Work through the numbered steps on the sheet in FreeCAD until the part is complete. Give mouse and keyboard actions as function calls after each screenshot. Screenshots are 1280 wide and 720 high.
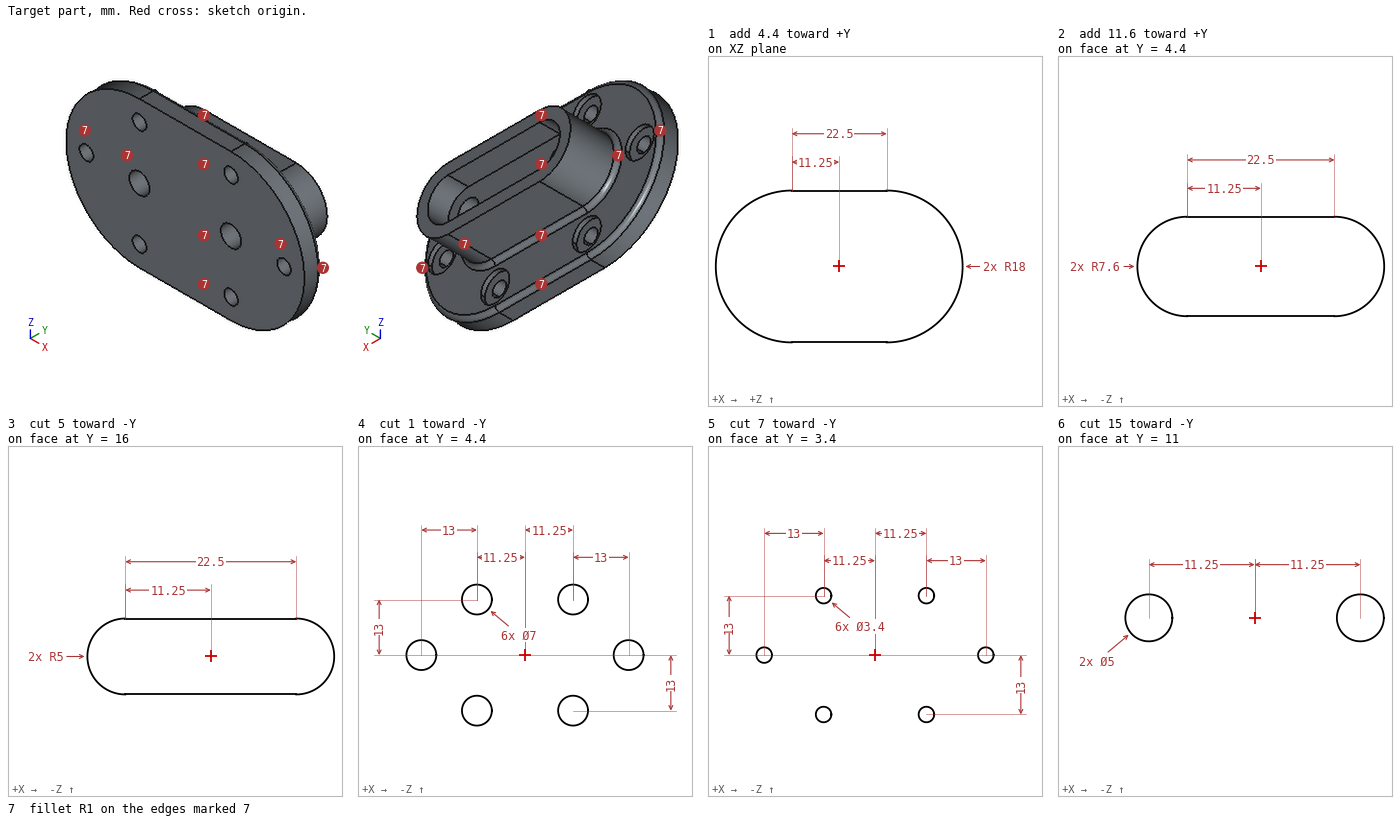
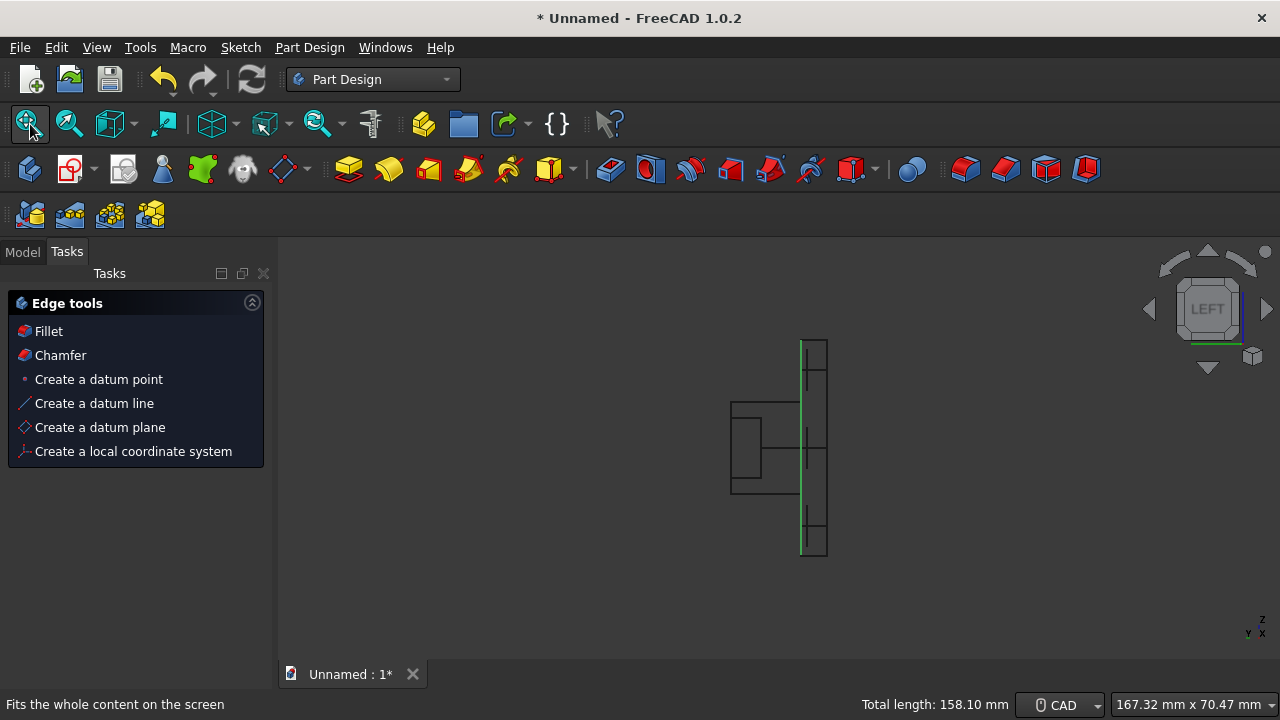
key(0)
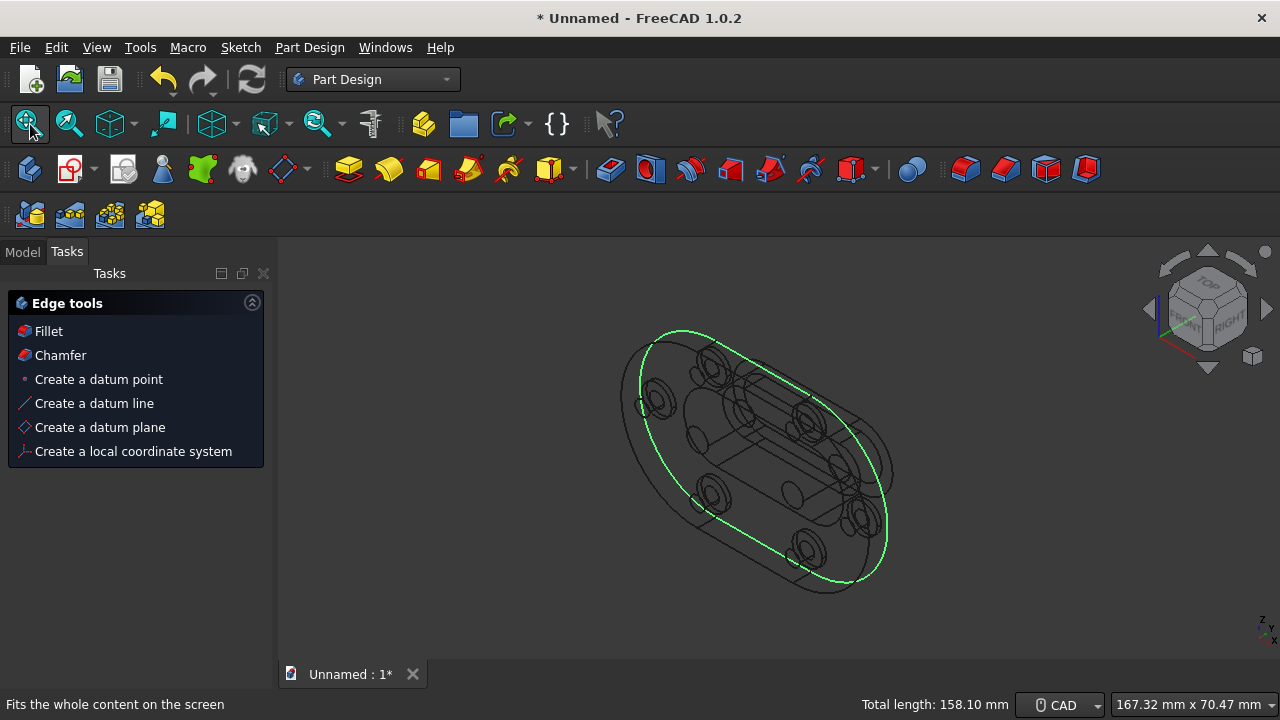
click(684, 410, ctrl)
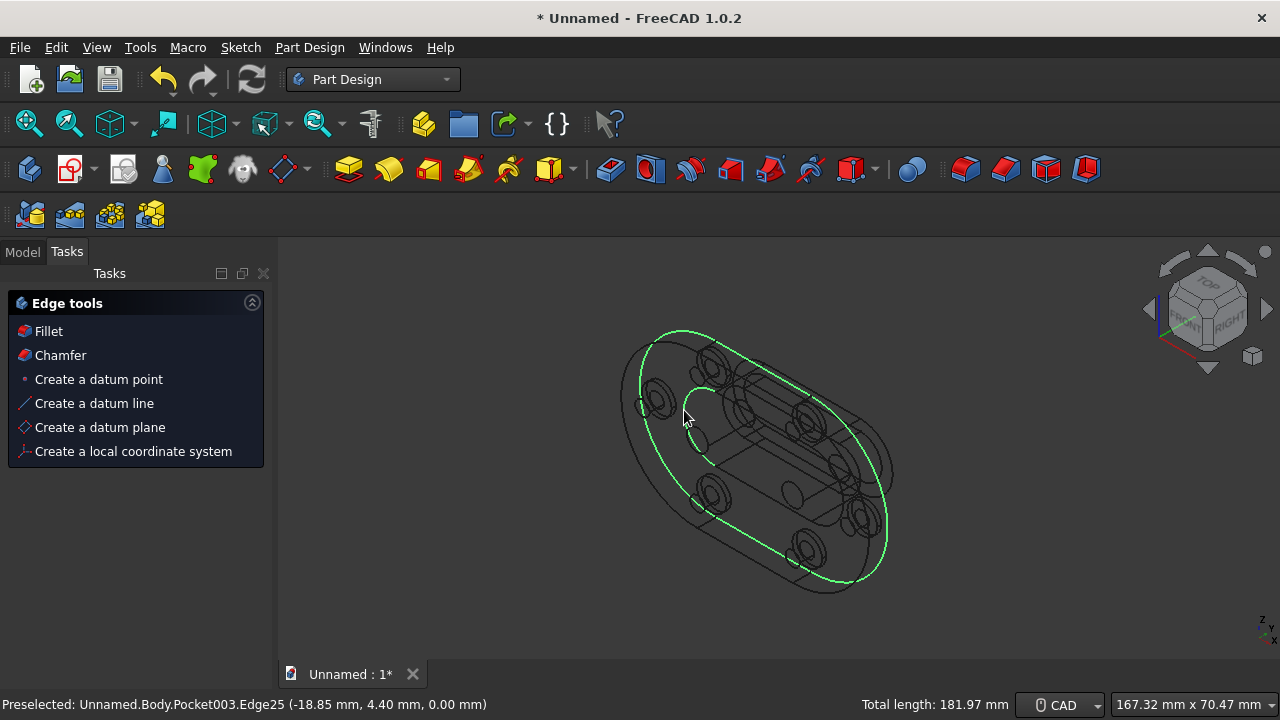
click(764, 419, ctrl)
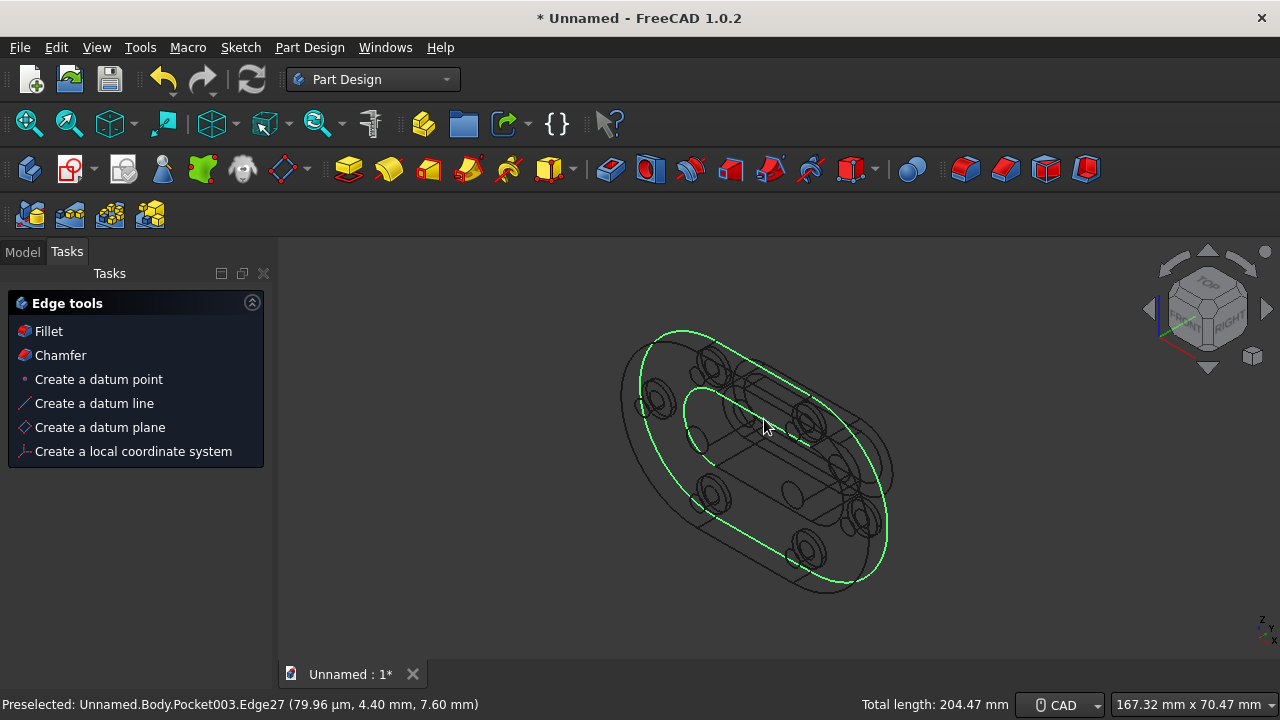
click(842, 489, ctrl)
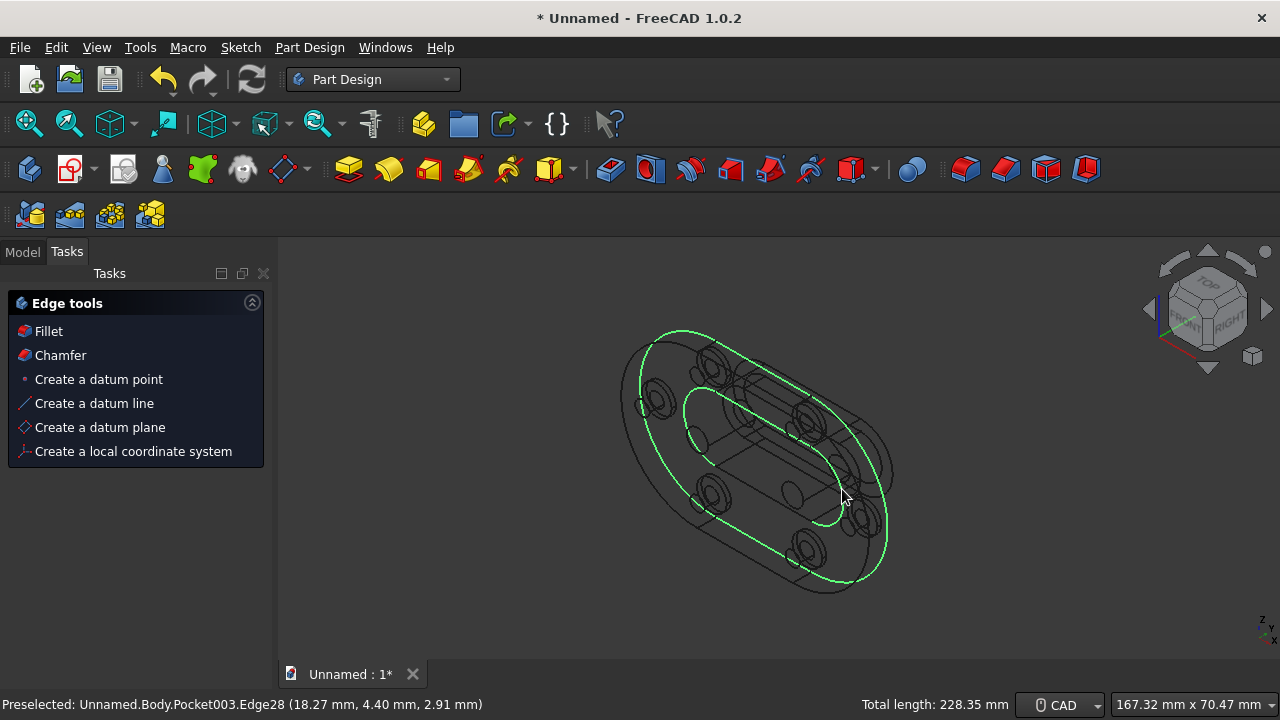
click(764, 493, ctrl)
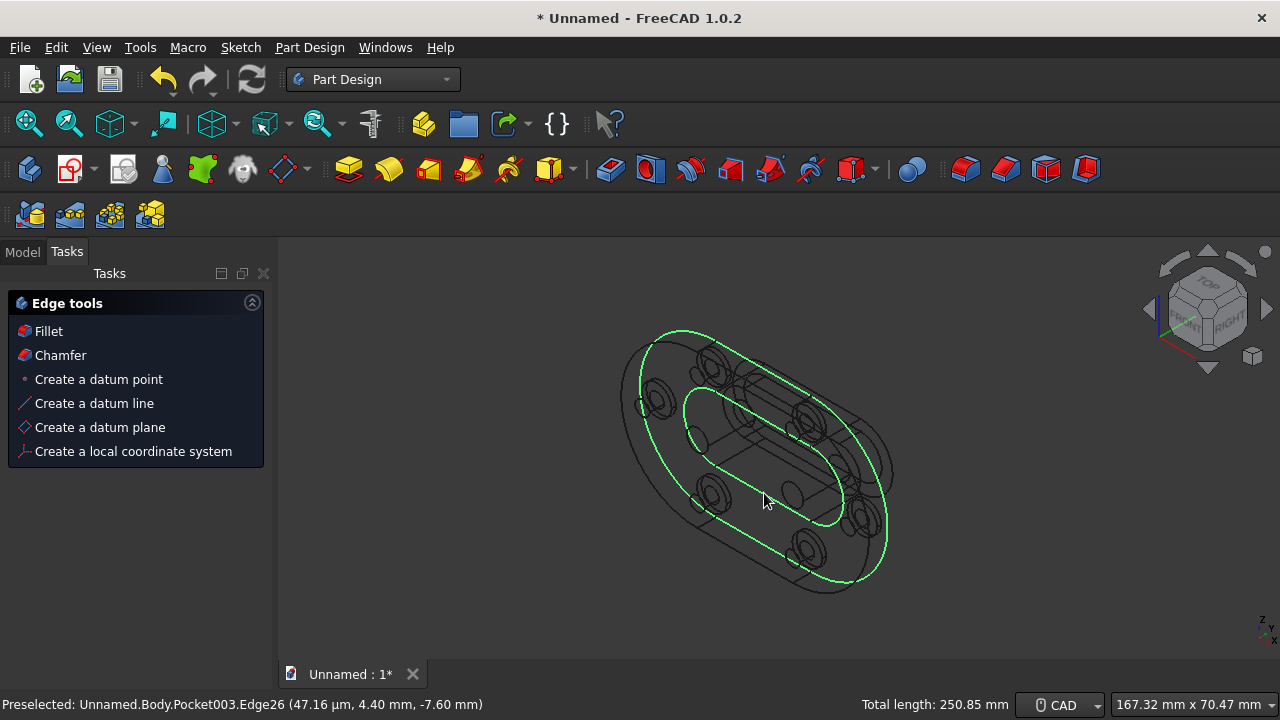
key(v)
key(1)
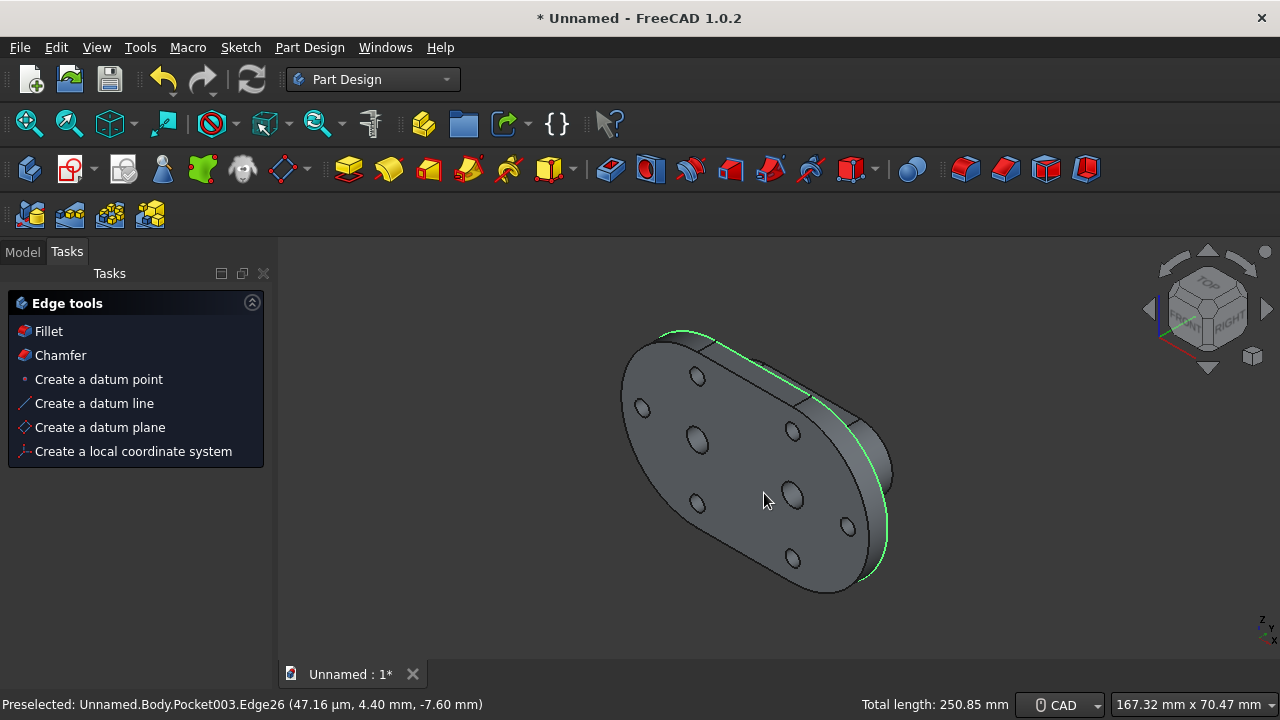
click(966, 170)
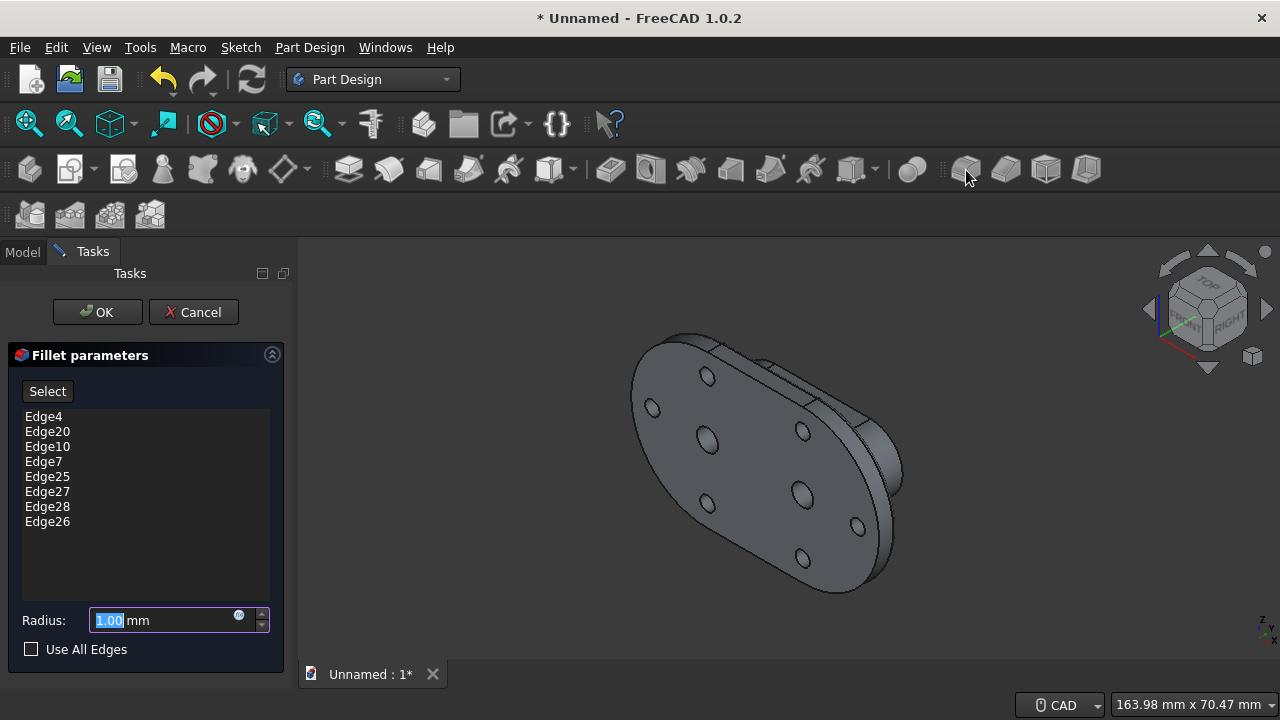
text(1)
key(Tab)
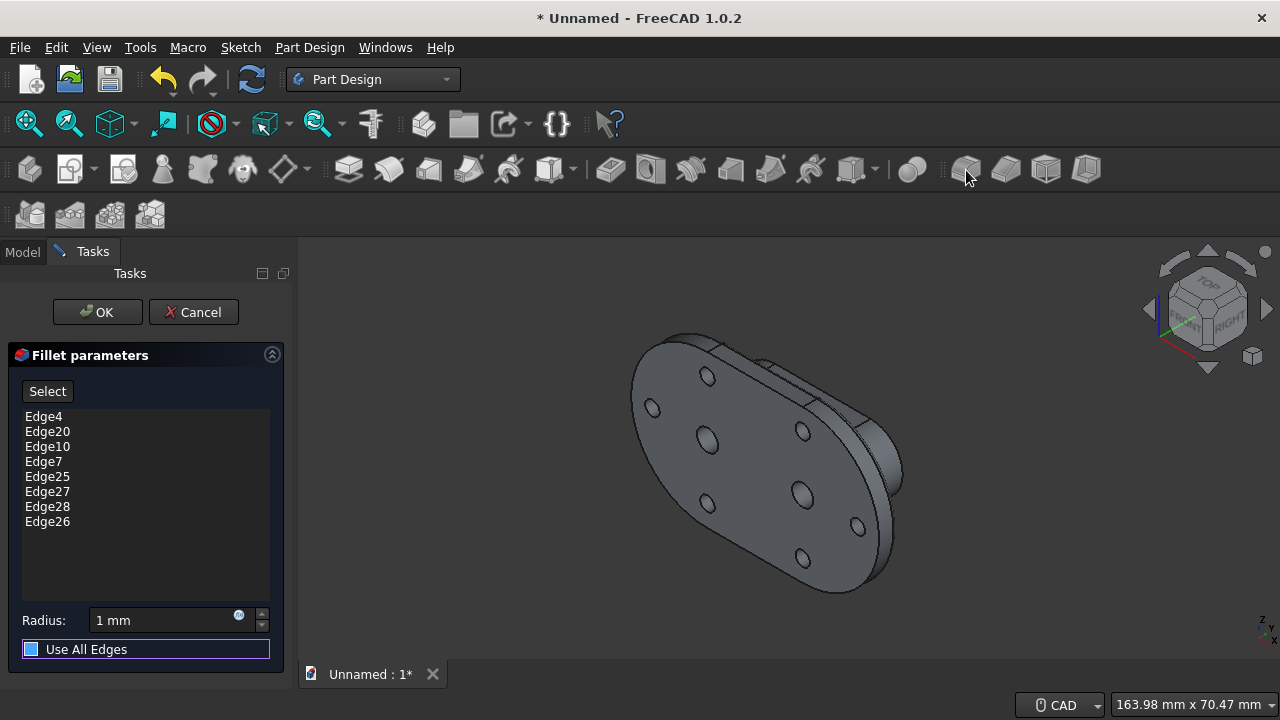
click(98, 312)